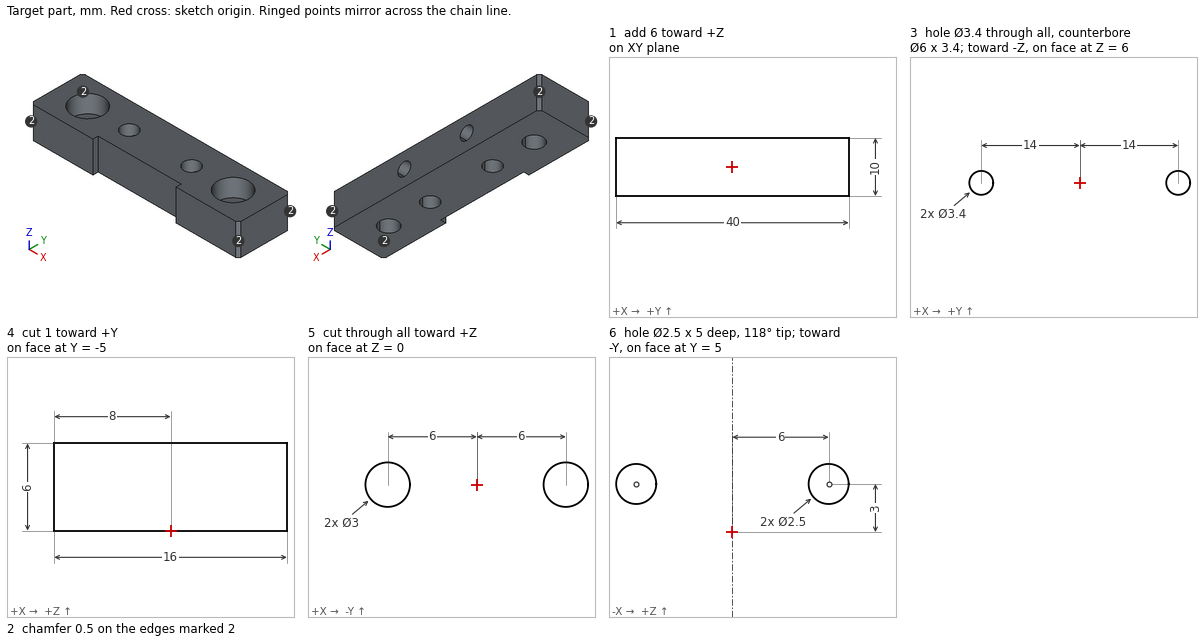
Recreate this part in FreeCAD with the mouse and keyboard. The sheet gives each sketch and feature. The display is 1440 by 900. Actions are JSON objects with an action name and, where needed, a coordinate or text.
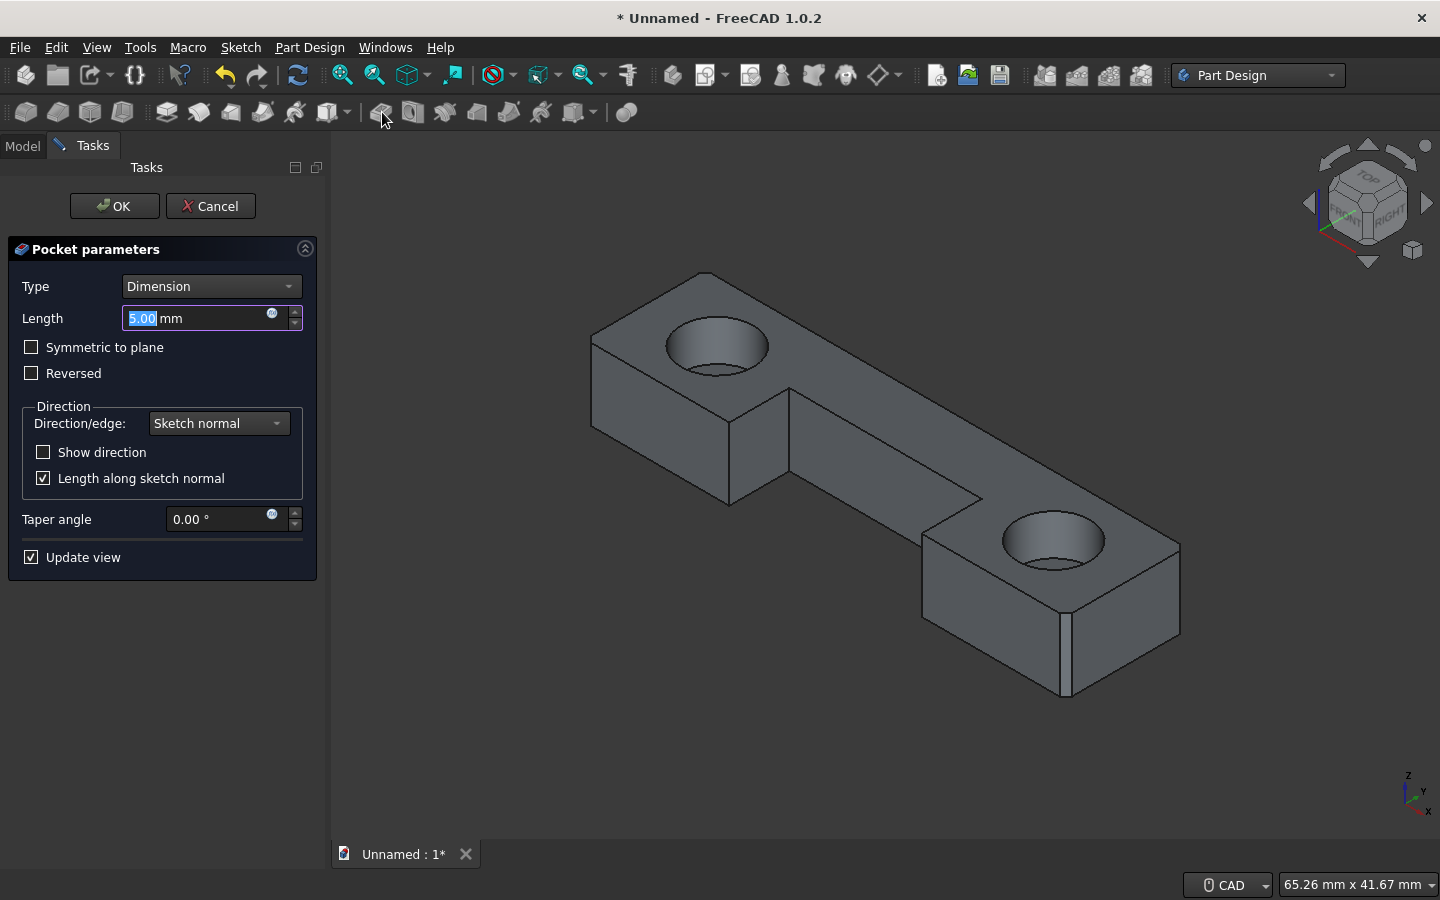
{"action": "type", "text": "1"}
{"action": "key", "text": "Tab"}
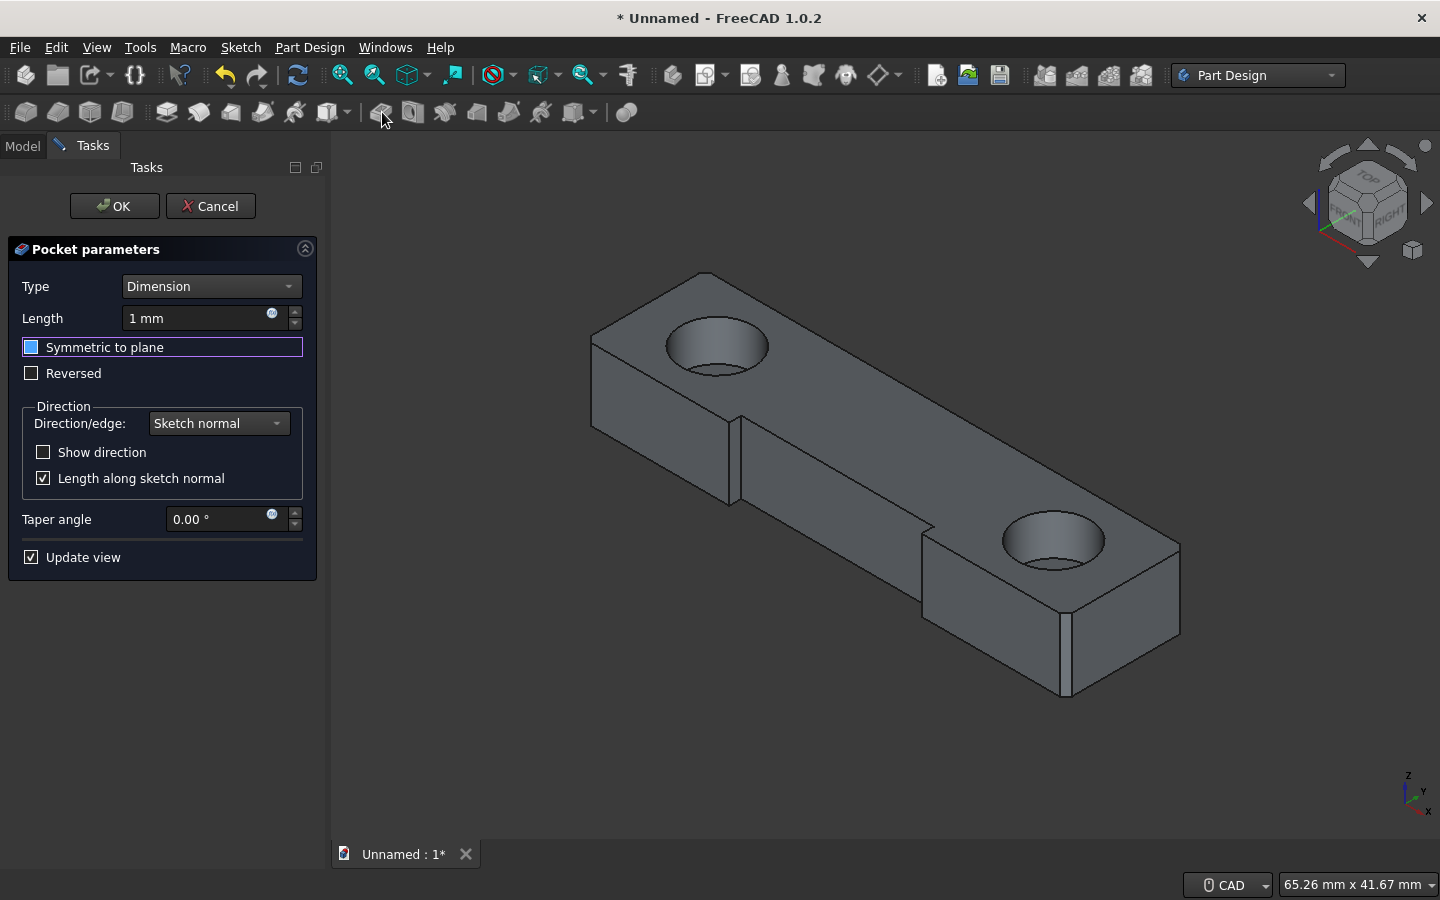
{"action": "left_click", "coordinate": [115, 206]}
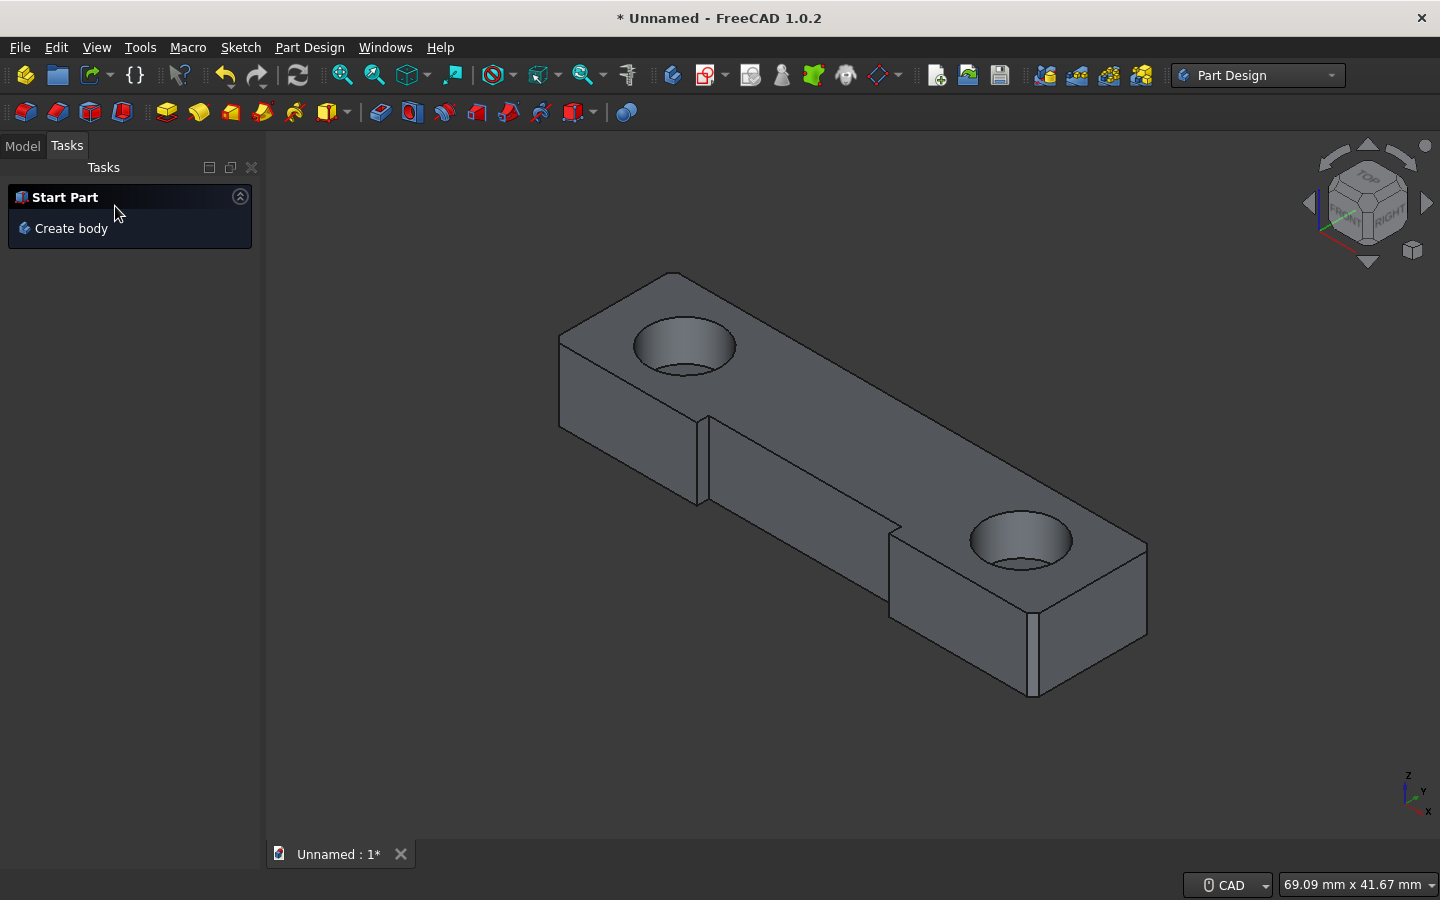
{"action": "key", "text": "5"}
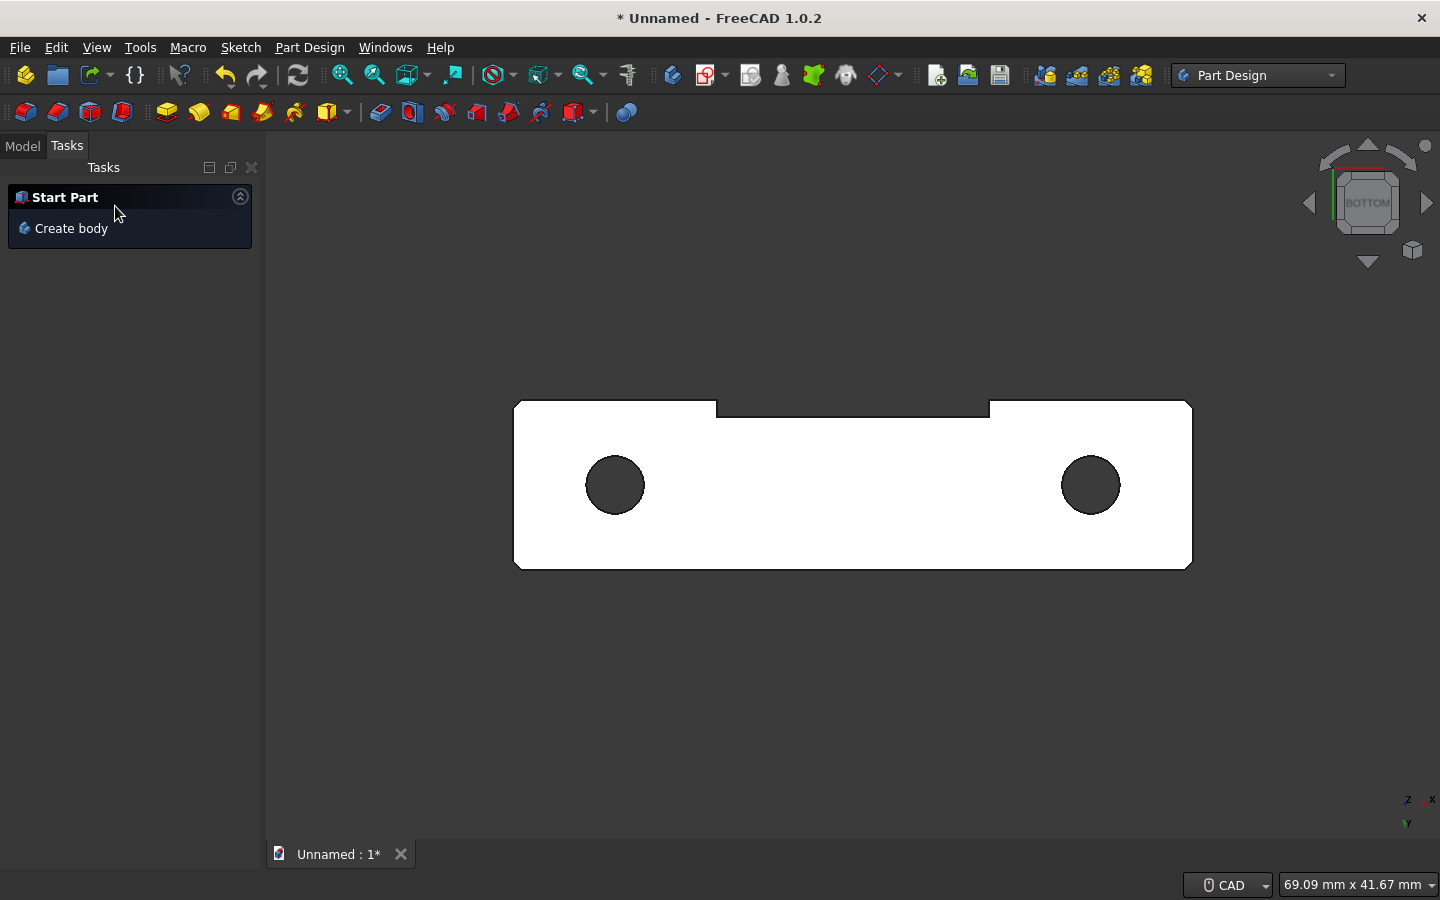
{"action": "left_click", "coordinate": [950, 484]}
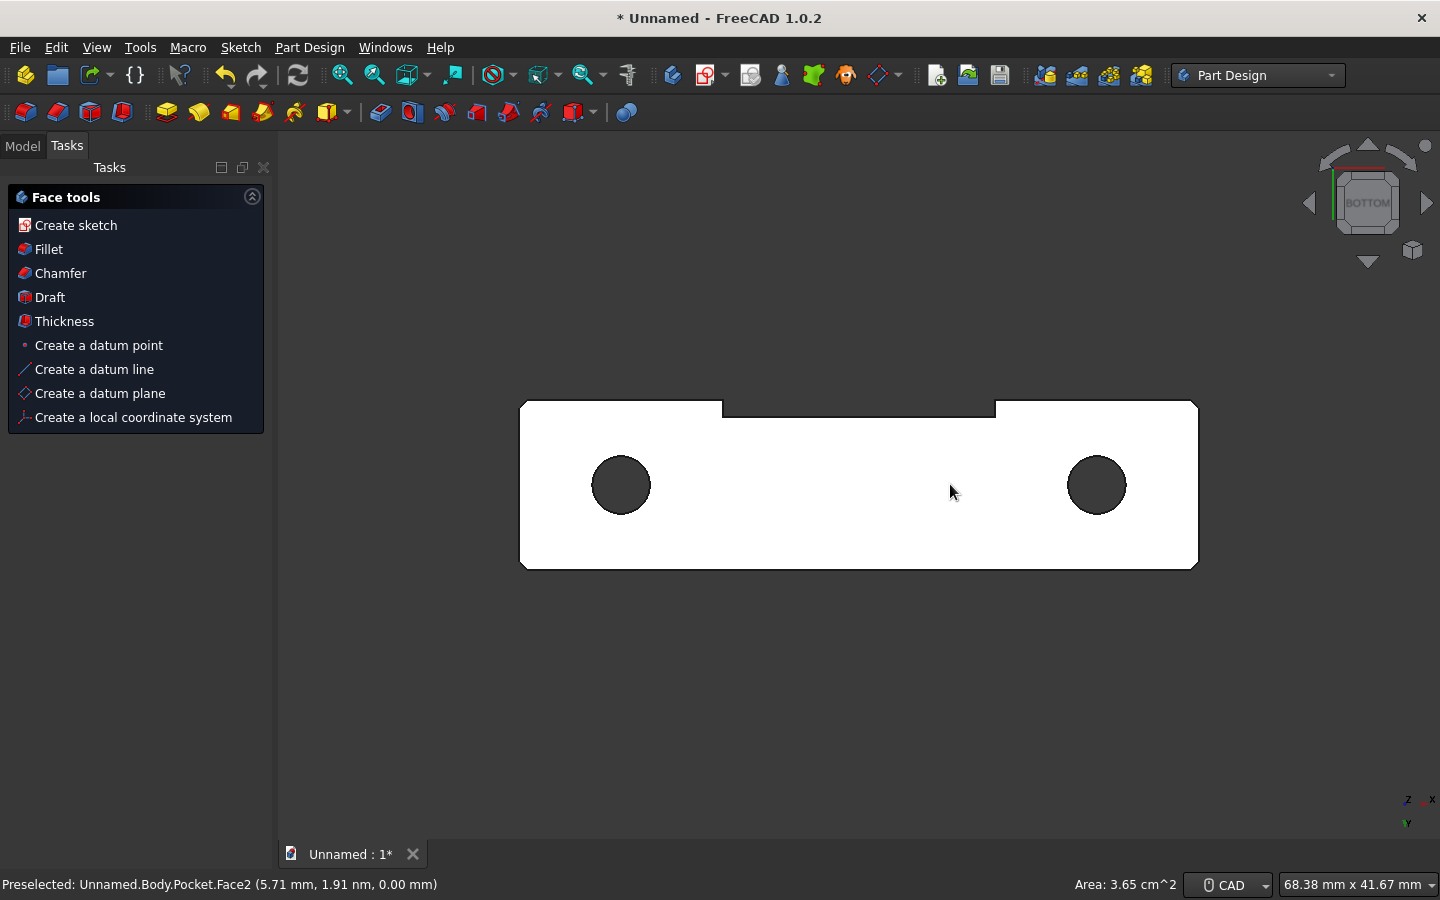
{"action": "left_click", "coordinate": [706, 76]}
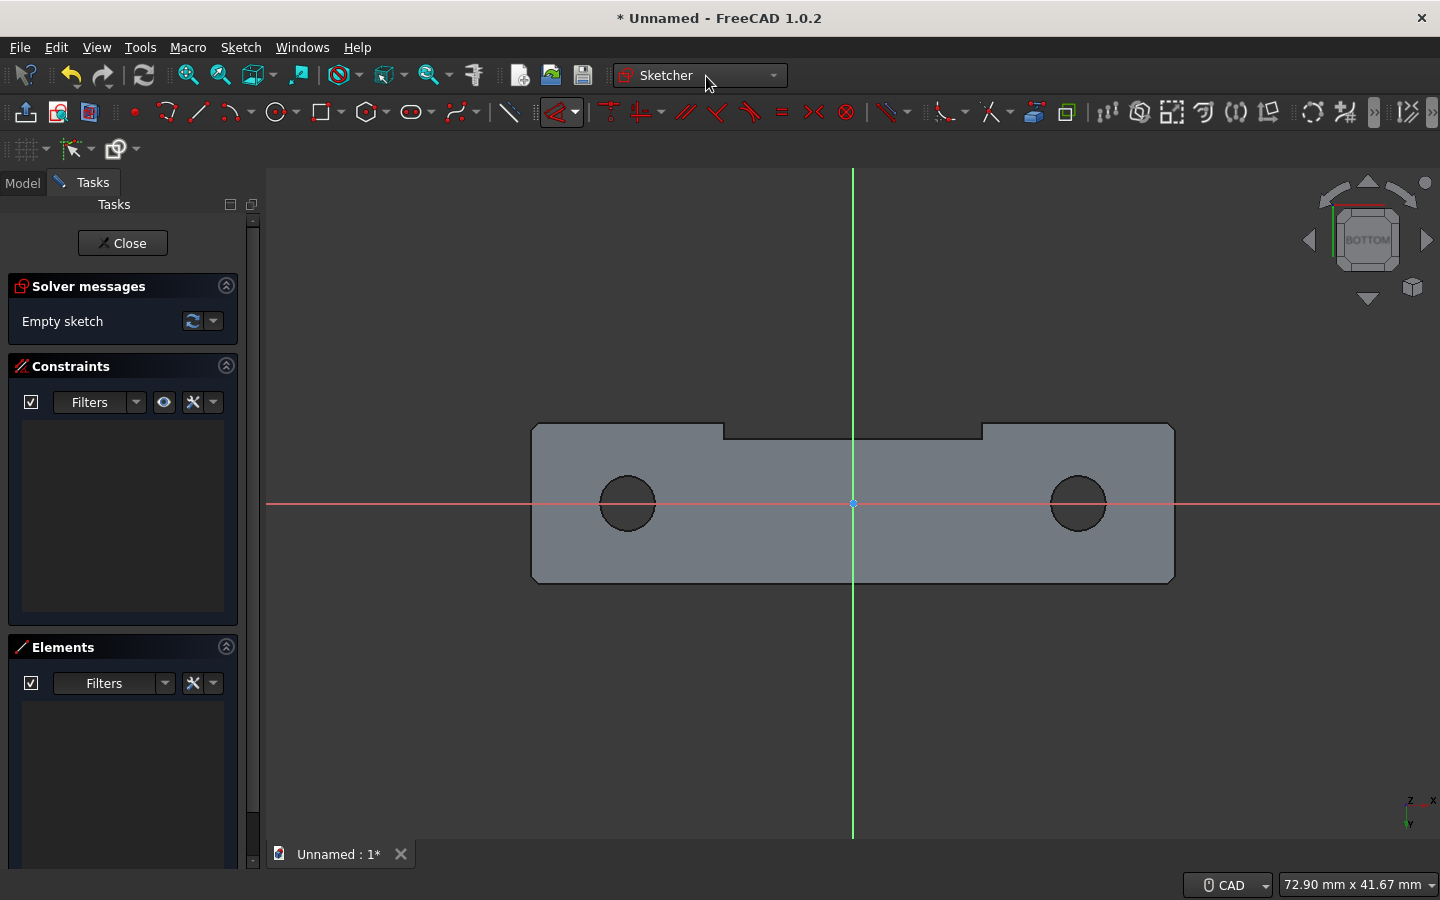
{"action": "scroll", "coordinate": [893, 503], "scroll_direction": "up", "scroll_amount": 5}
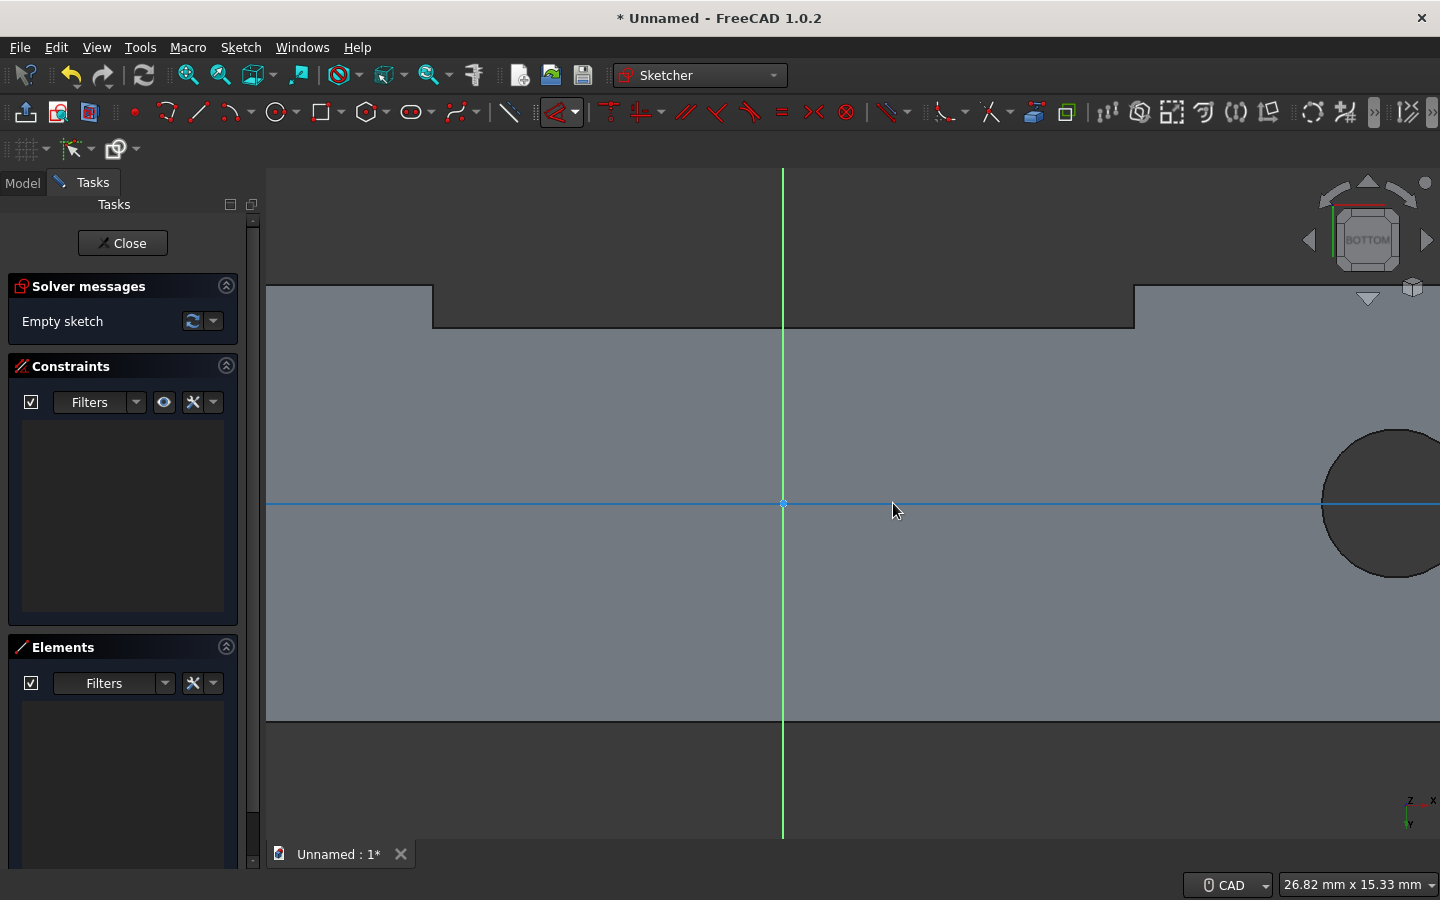
{"action": "left_click", "coordinate": [276, 112]}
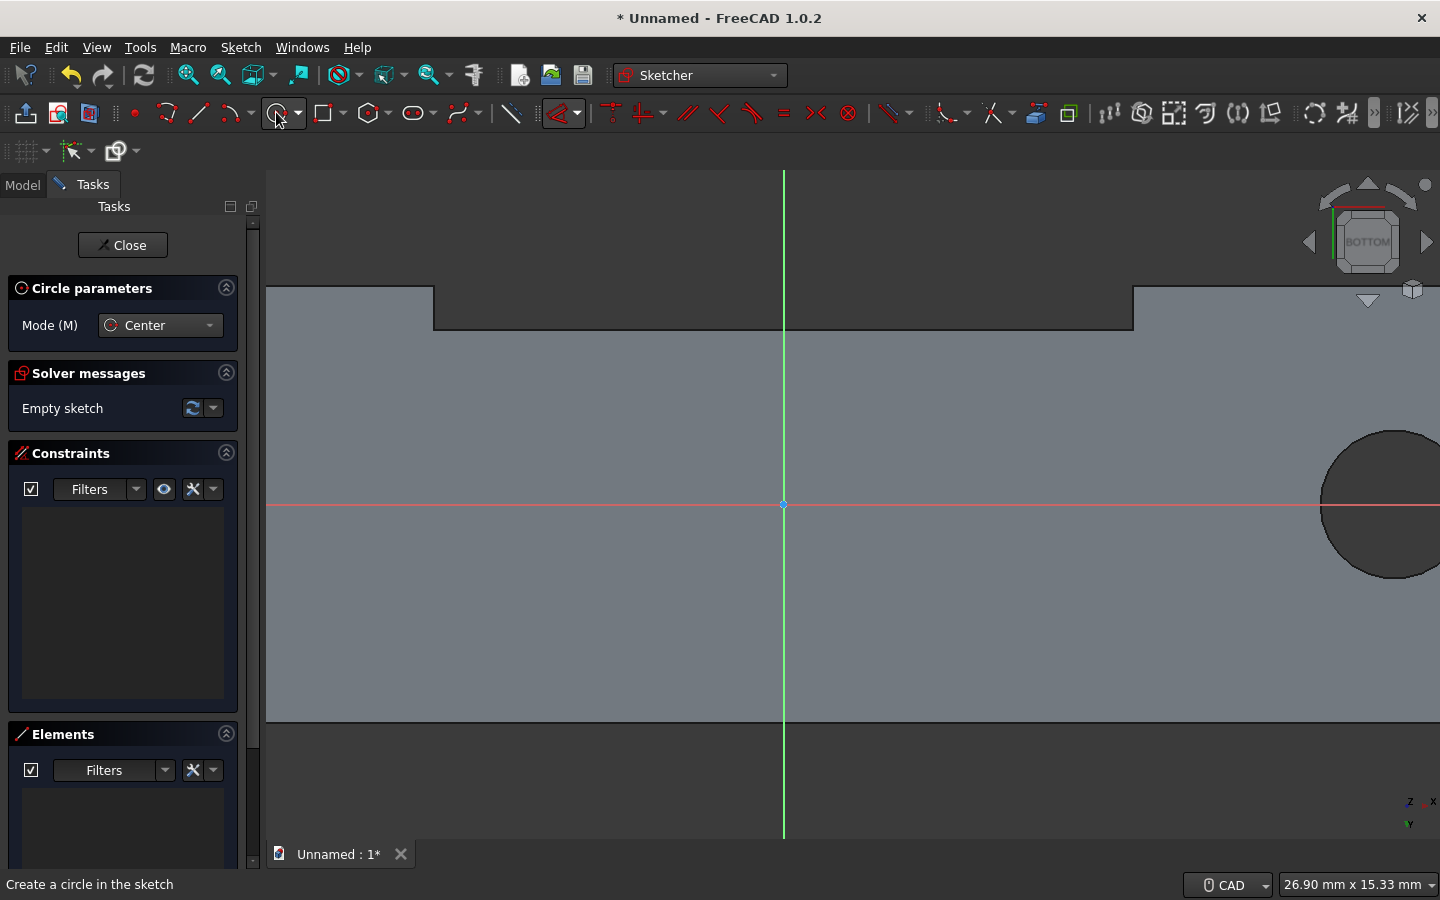
{"action": "left_click", "coordinate": [522, 504]}
{"action": "mouse_move", "coordinate": [568, 458]}